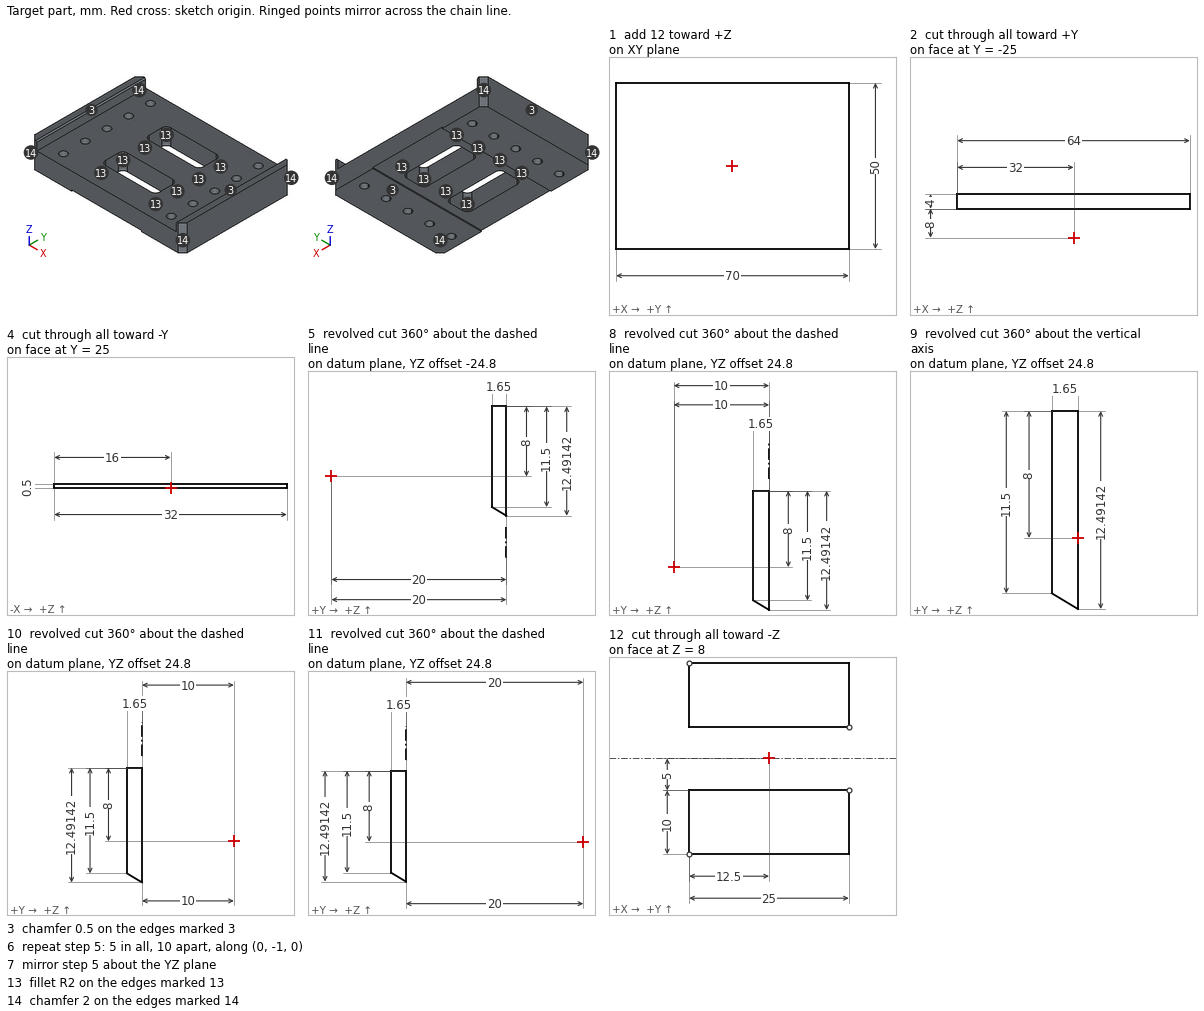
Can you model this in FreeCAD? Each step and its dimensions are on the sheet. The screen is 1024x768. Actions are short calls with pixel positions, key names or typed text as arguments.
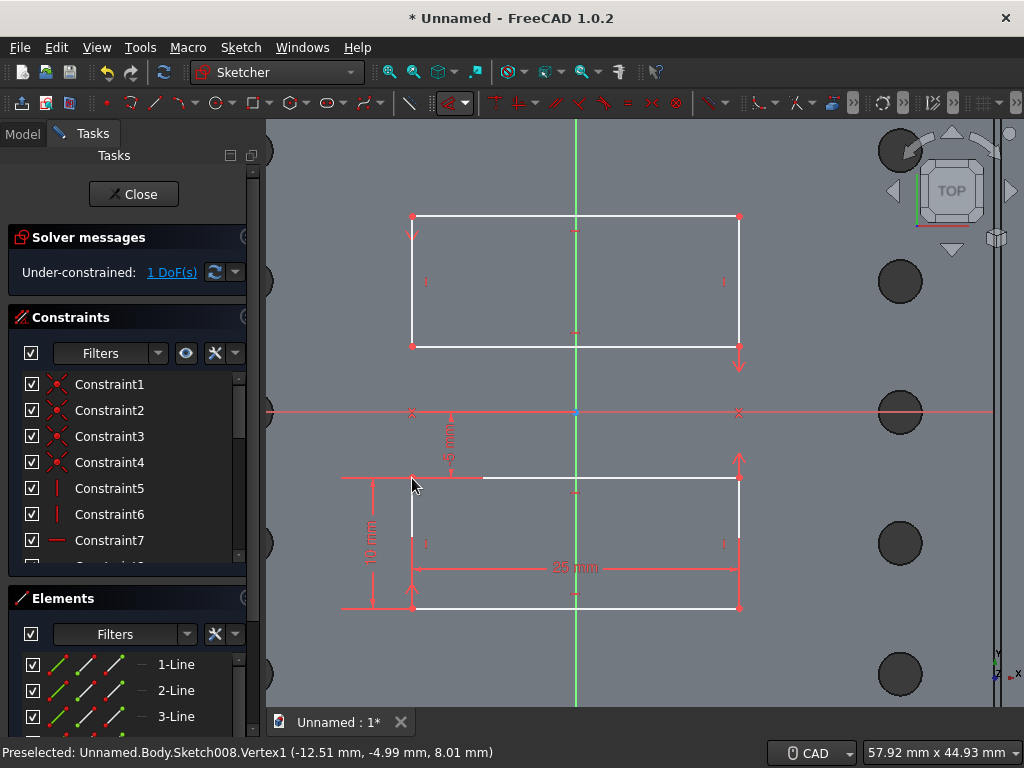
click(412, 478)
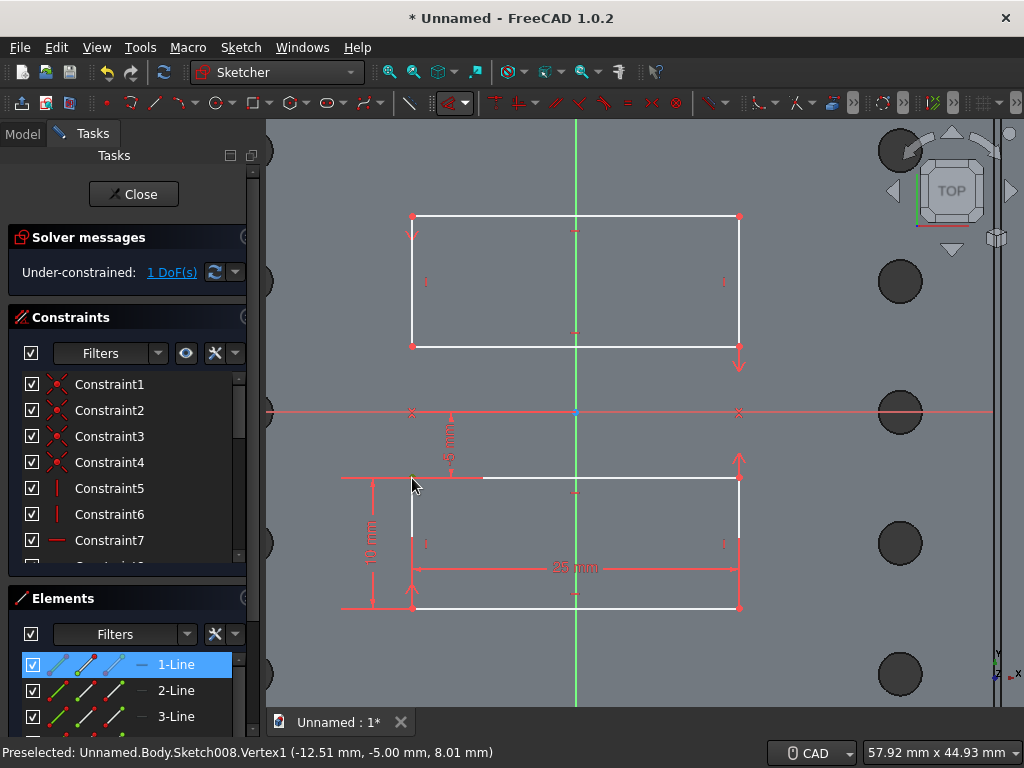
key(l)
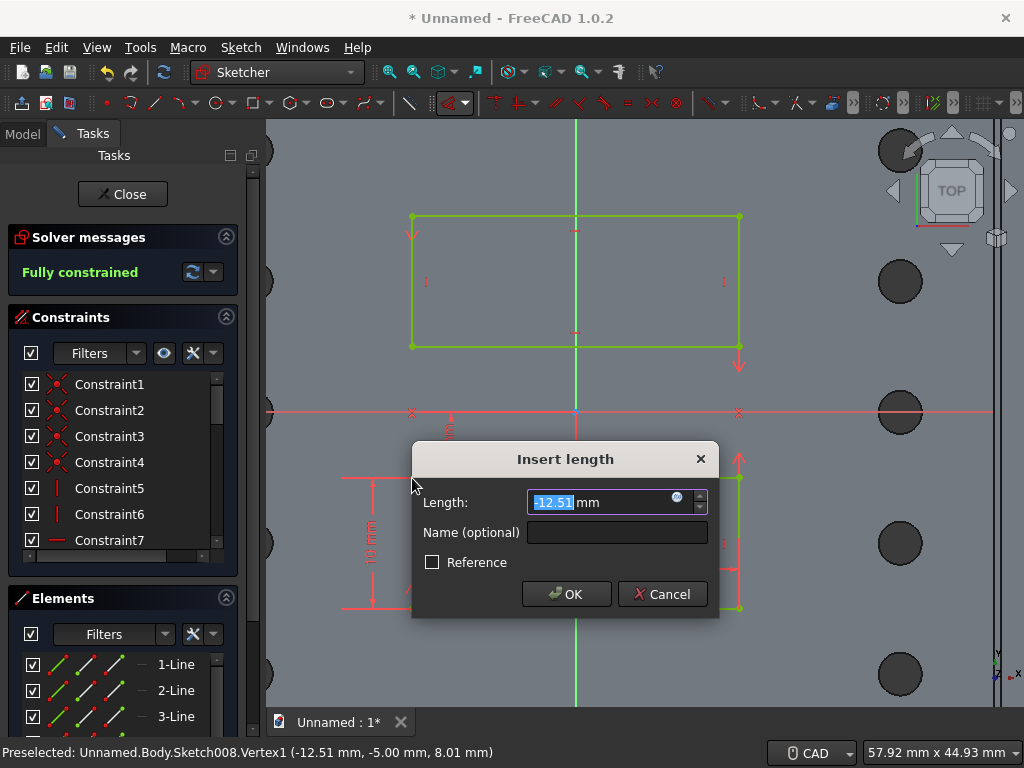
text(-12.5)
key(Return)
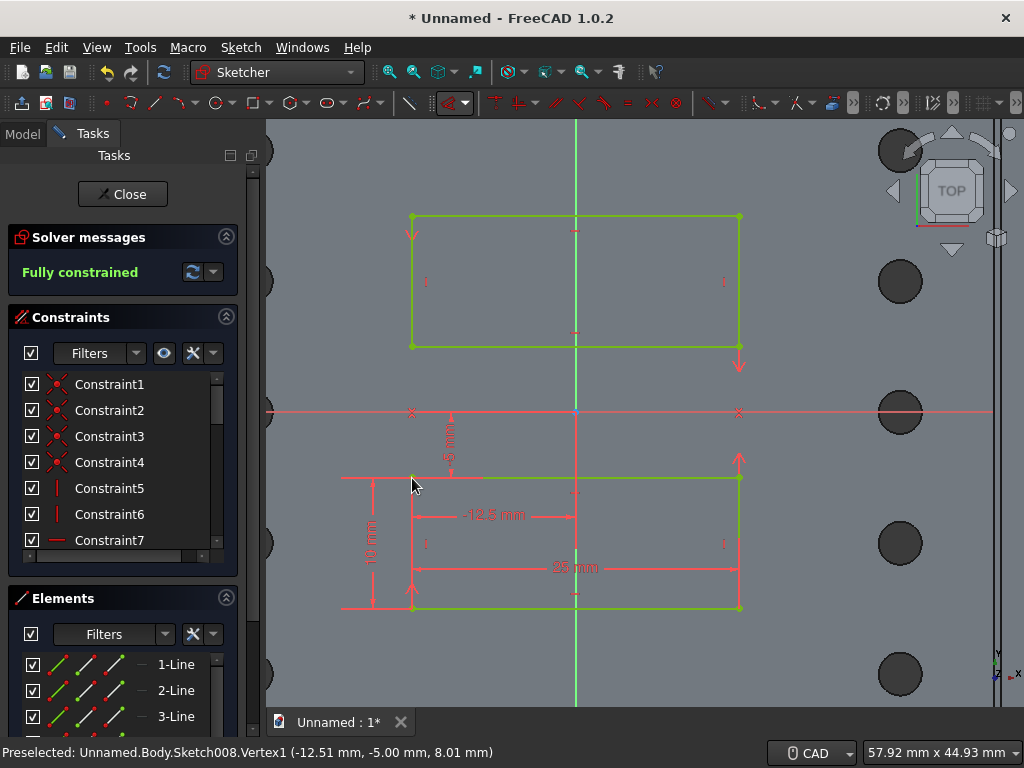
click(123, 194)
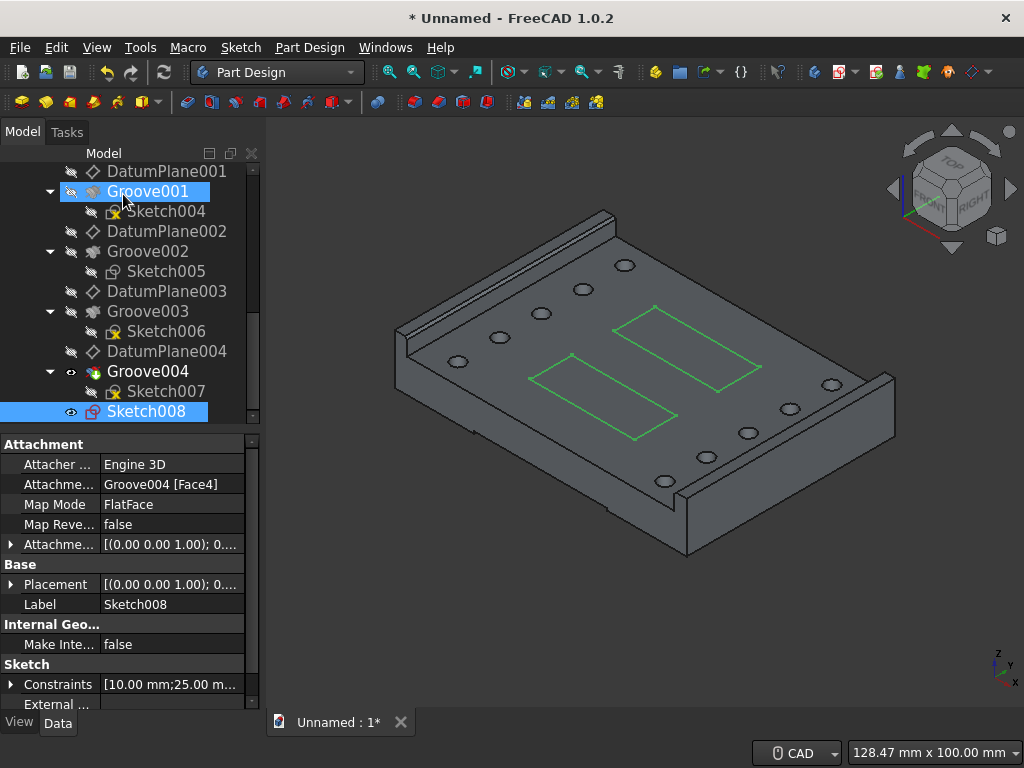
click(188, 102)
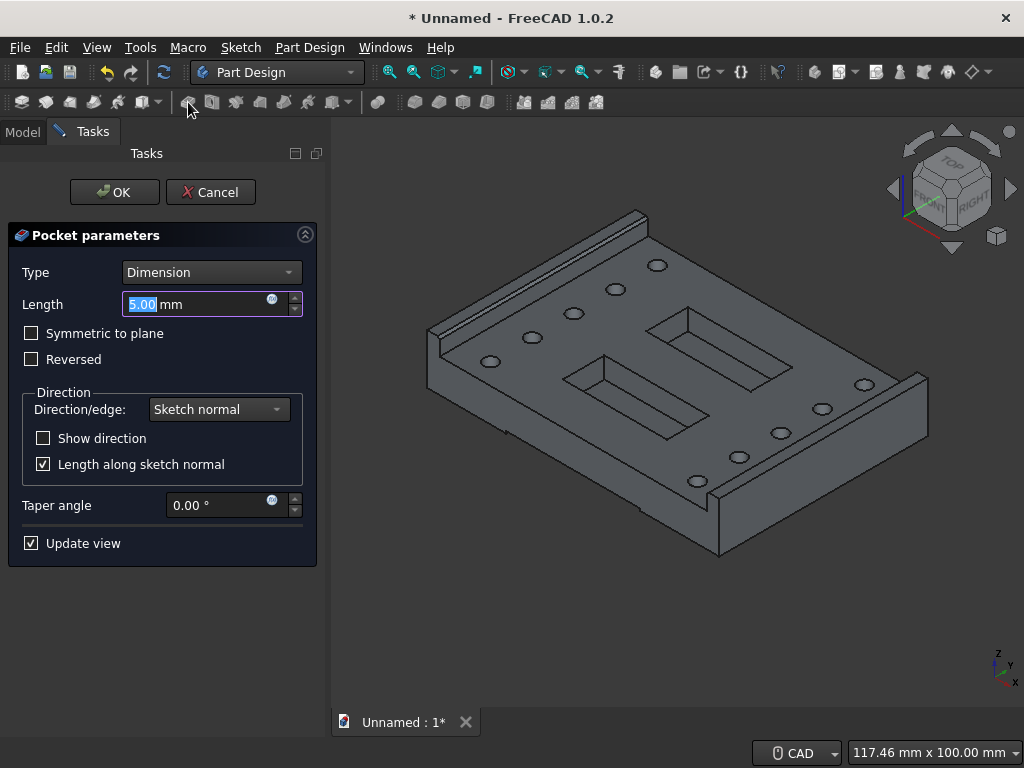
click(212, 272)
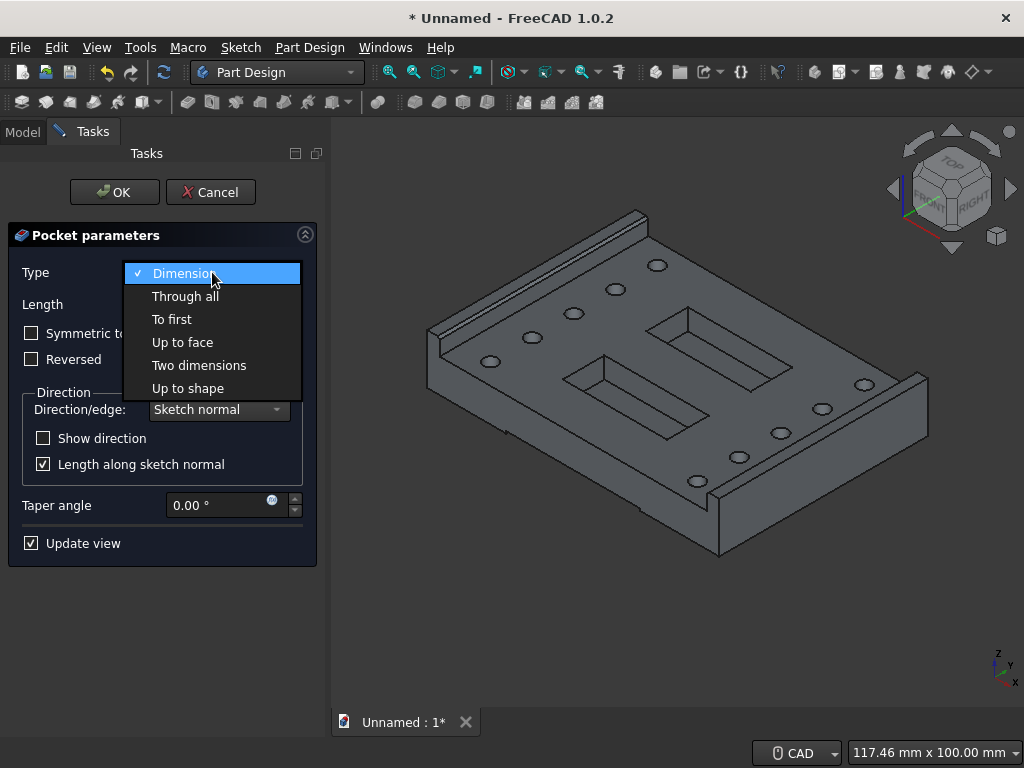
click(212, 296)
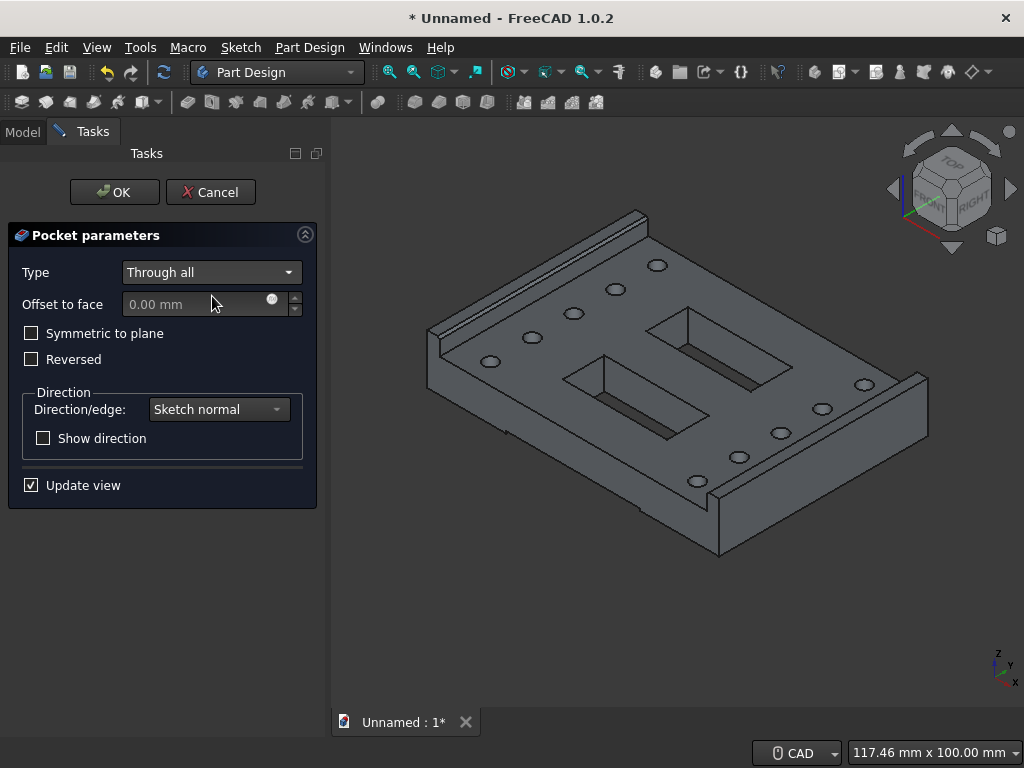
click(115, 192)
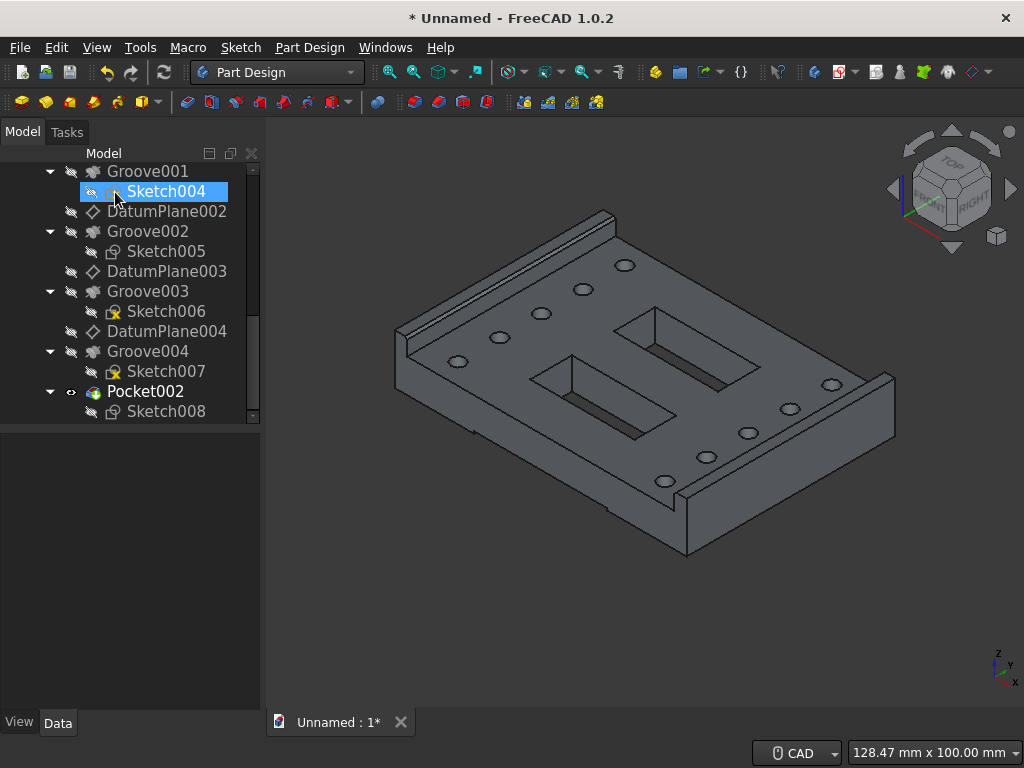
key(2)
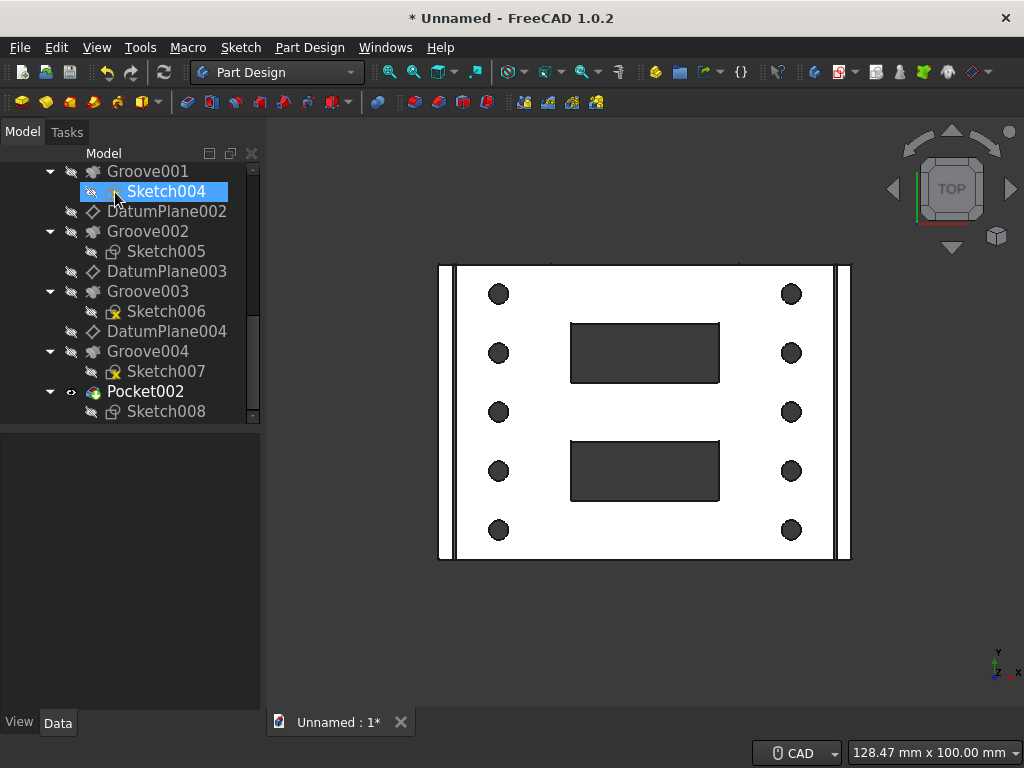
key(0)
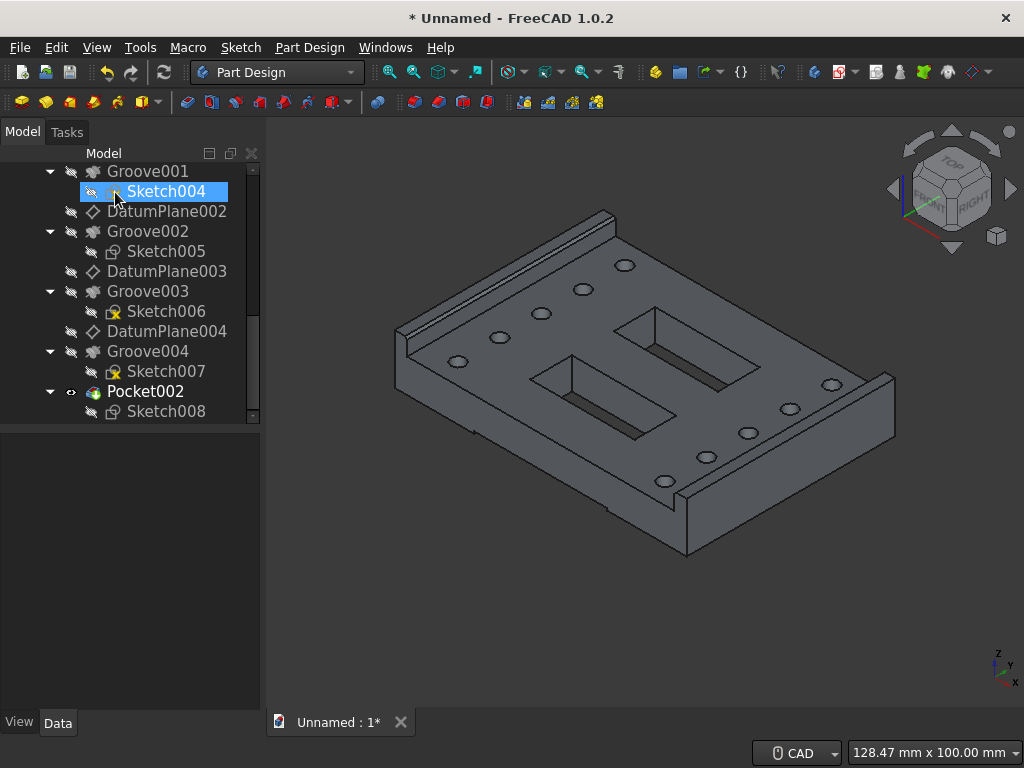
key(1)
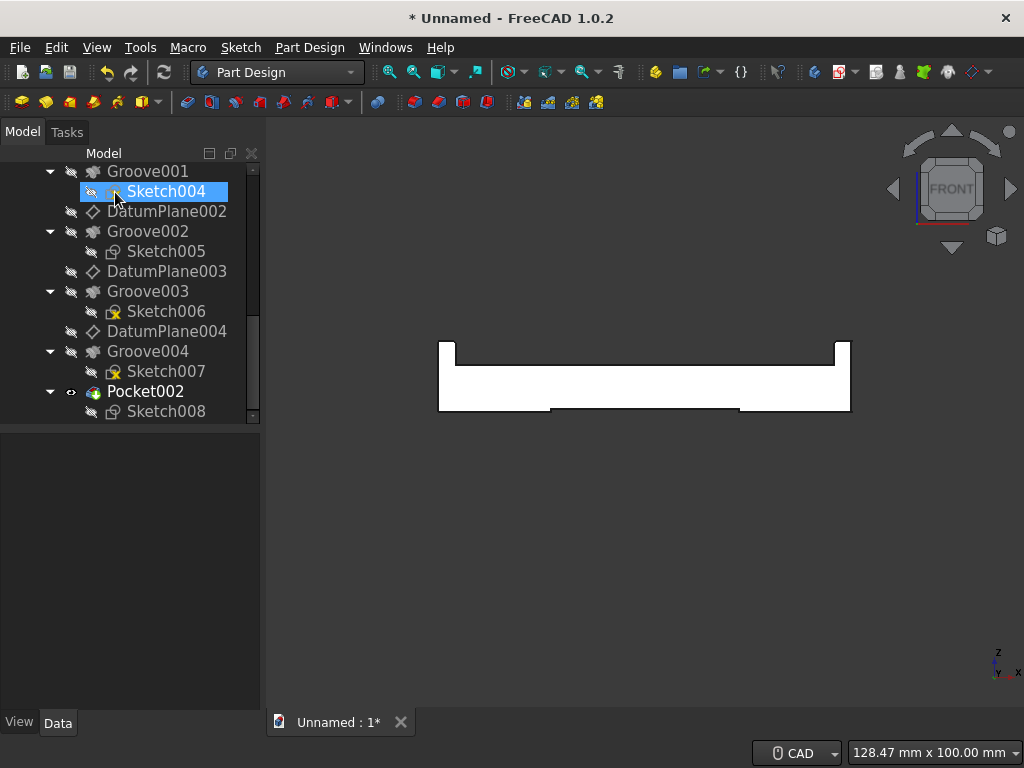
key(3)